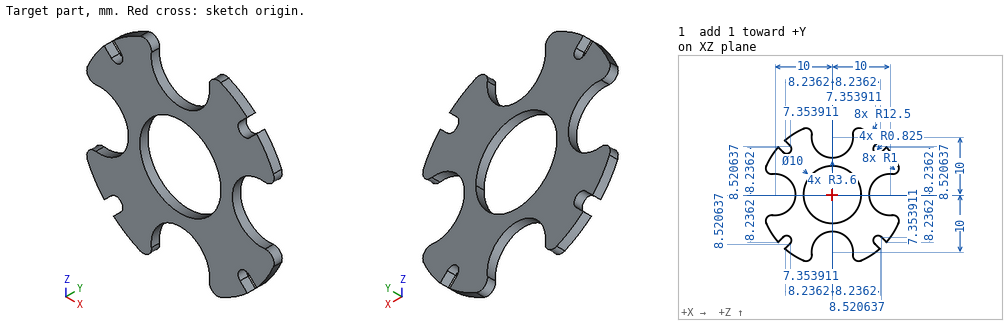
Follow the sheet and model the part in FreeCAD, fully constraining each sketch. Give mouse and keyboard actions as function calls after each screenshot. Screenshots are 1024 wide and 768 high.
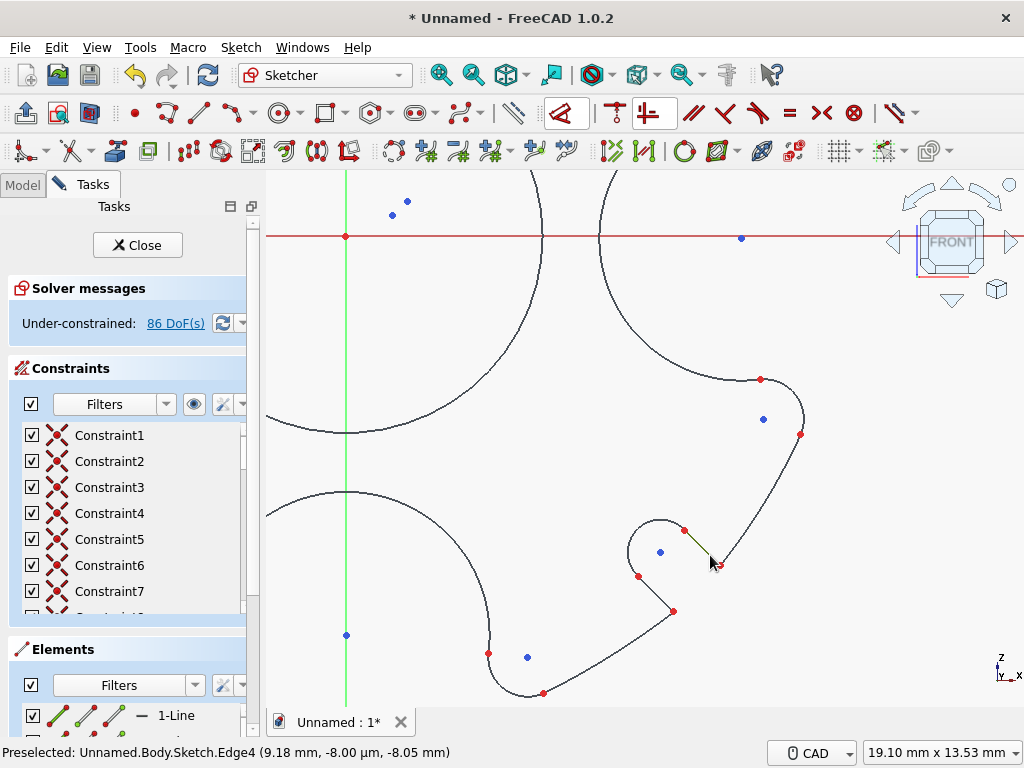
click(656, 520)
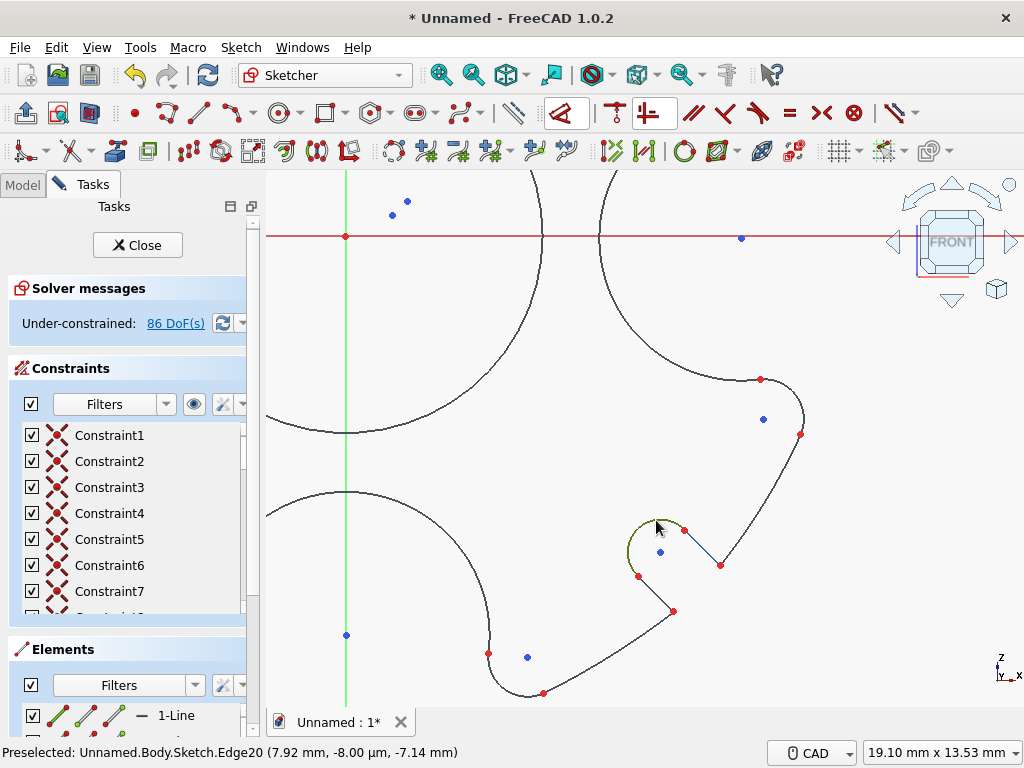
click(758, 114)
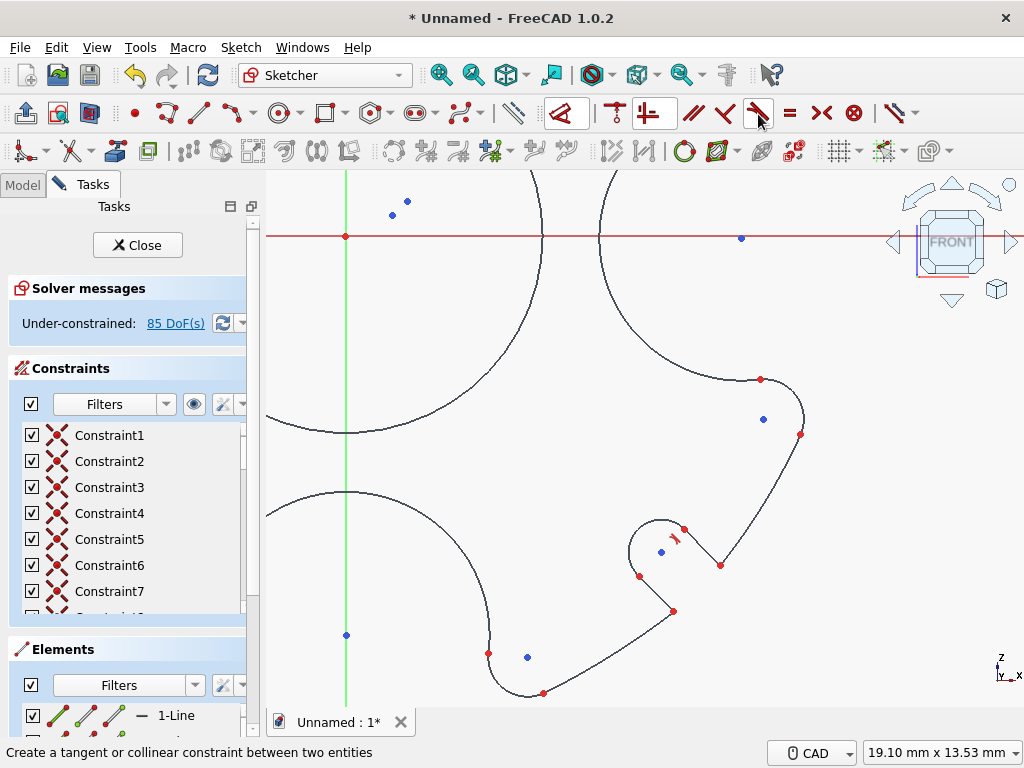
click(650, 587)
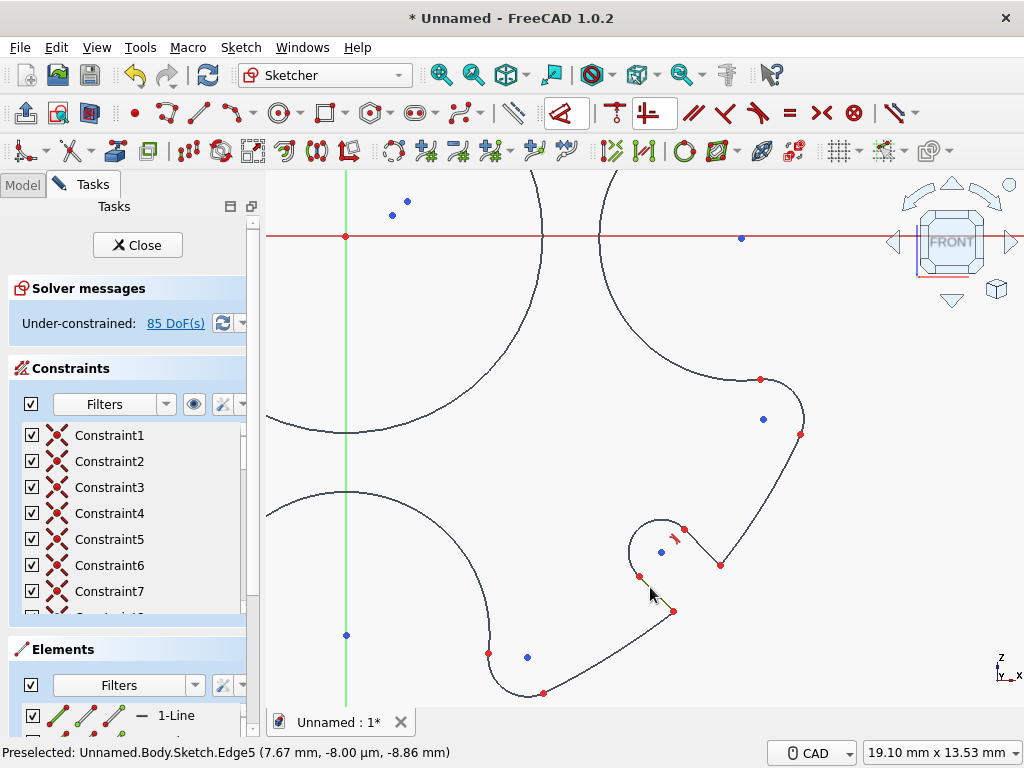
click(656, 520)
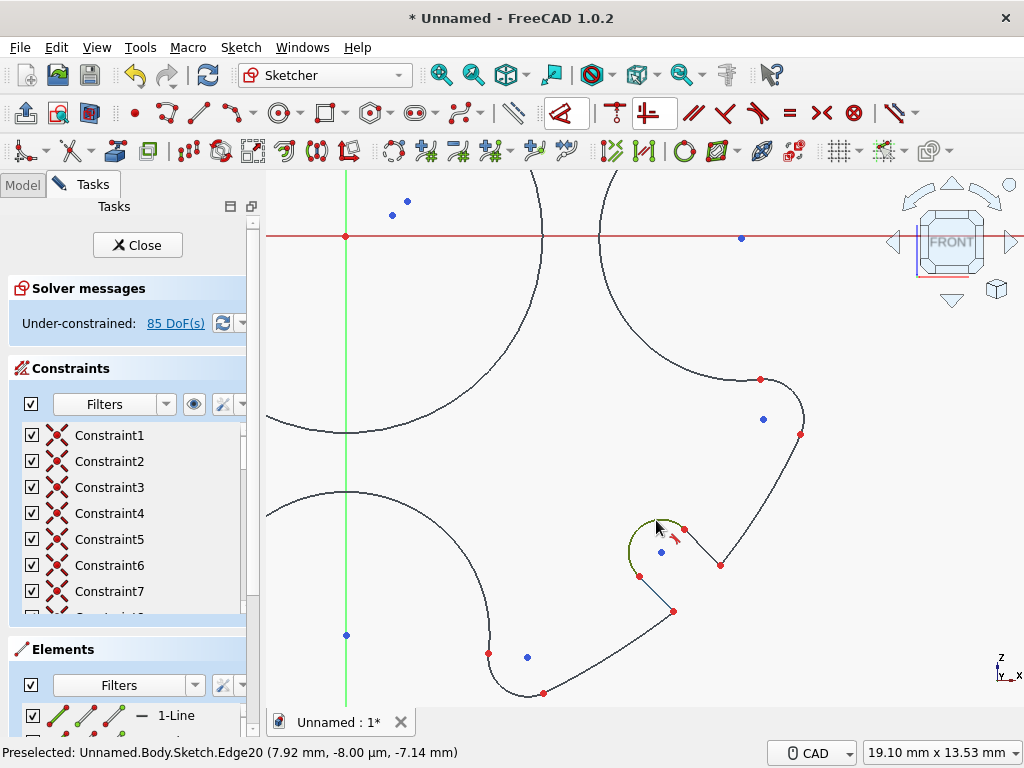
key(t)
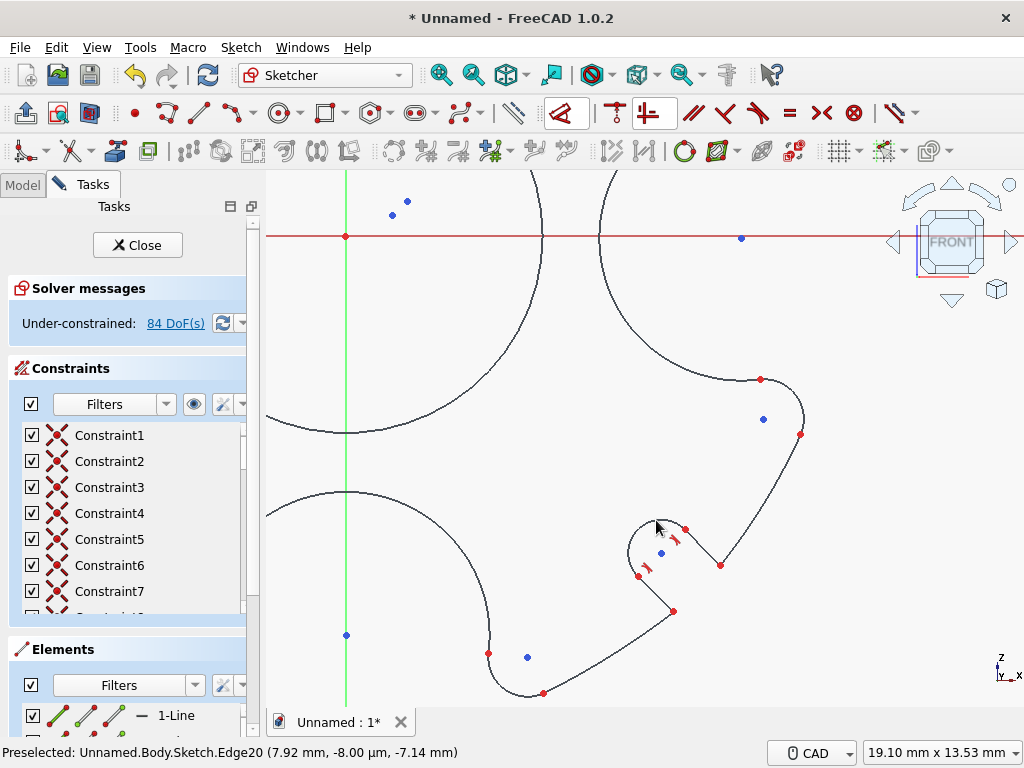
scroll(711, 556, down, 5)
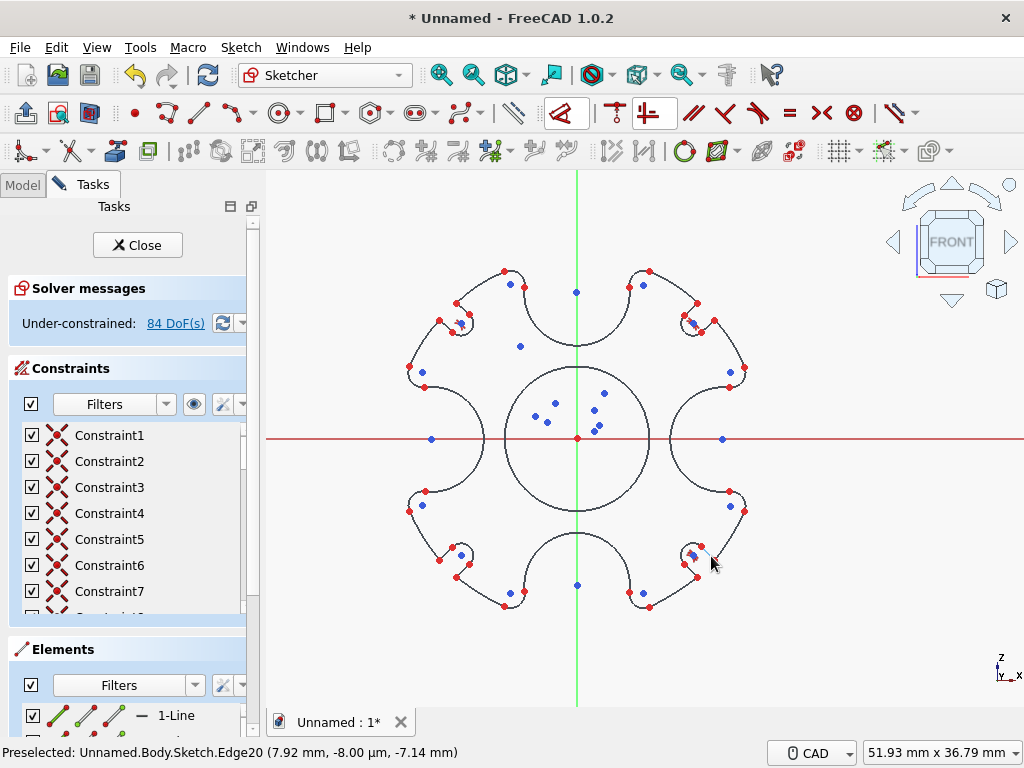
scroll(461, 573, up, 5)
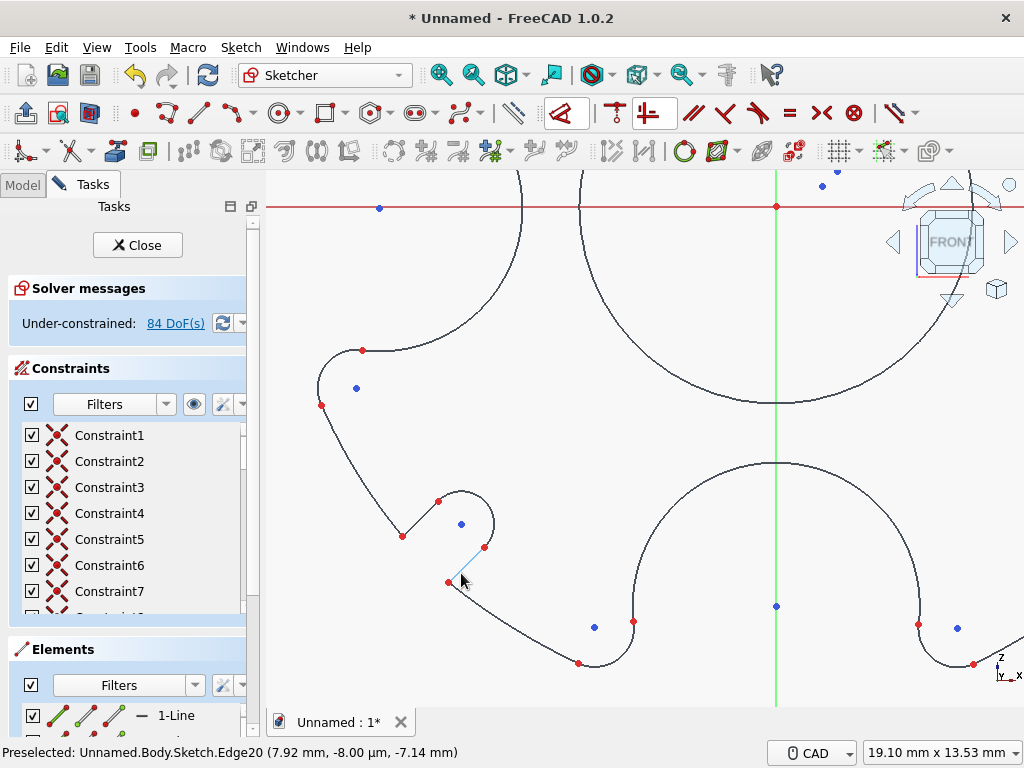
click(460, 572)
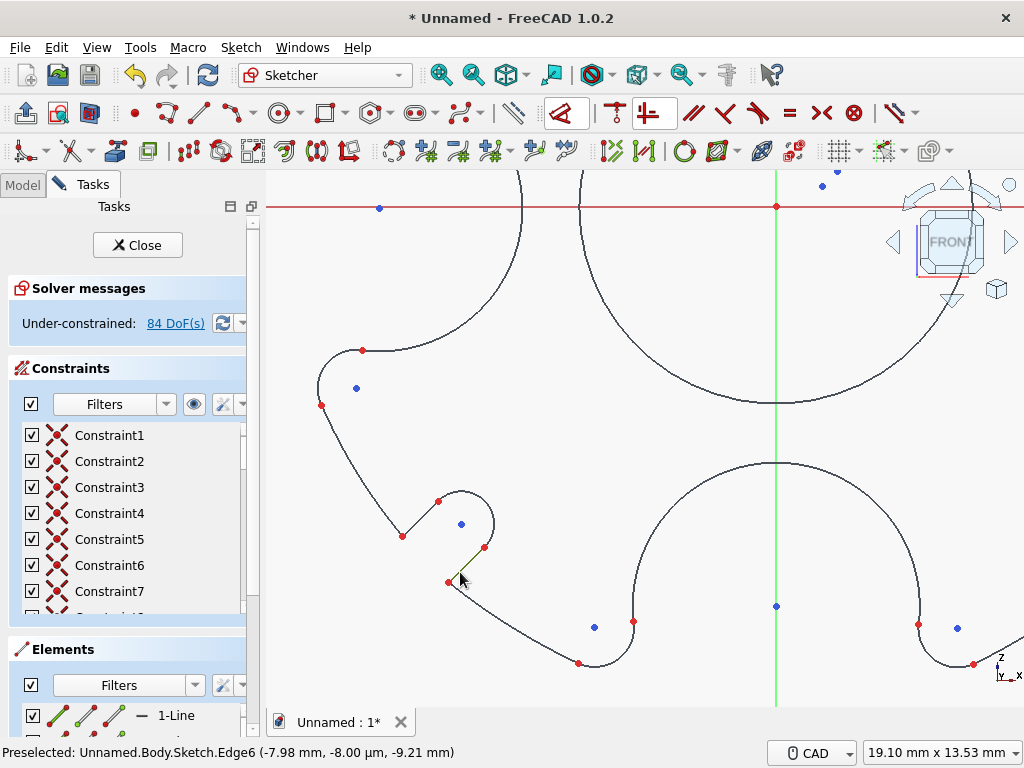
click(494, 519)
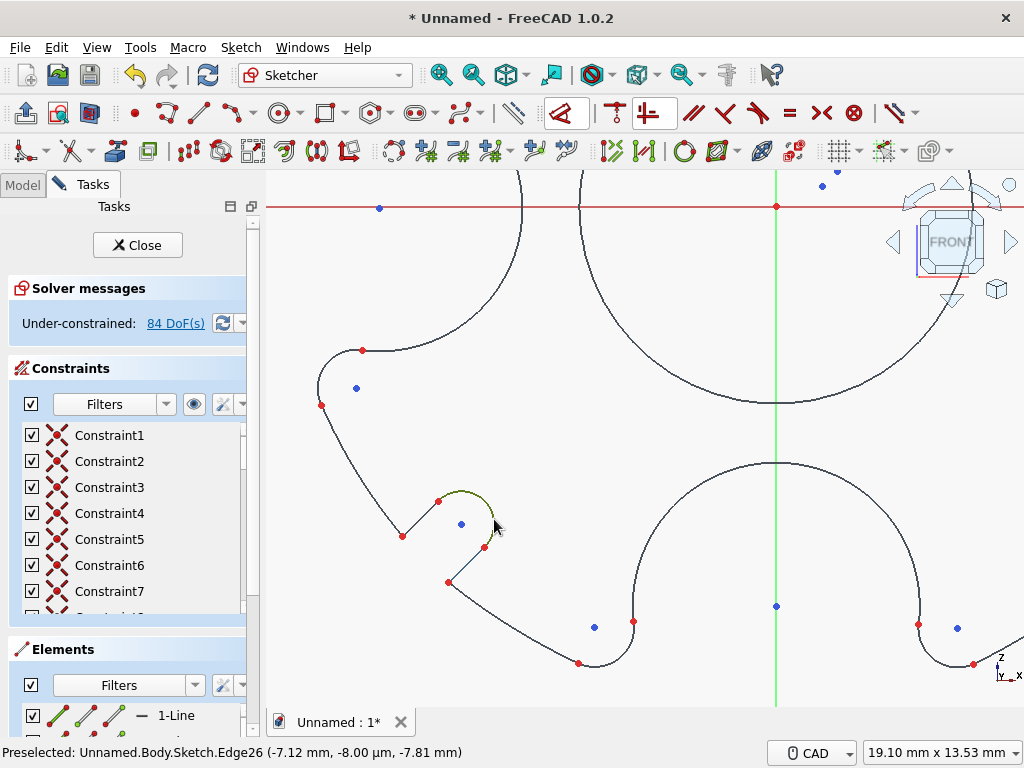
click(758, 114)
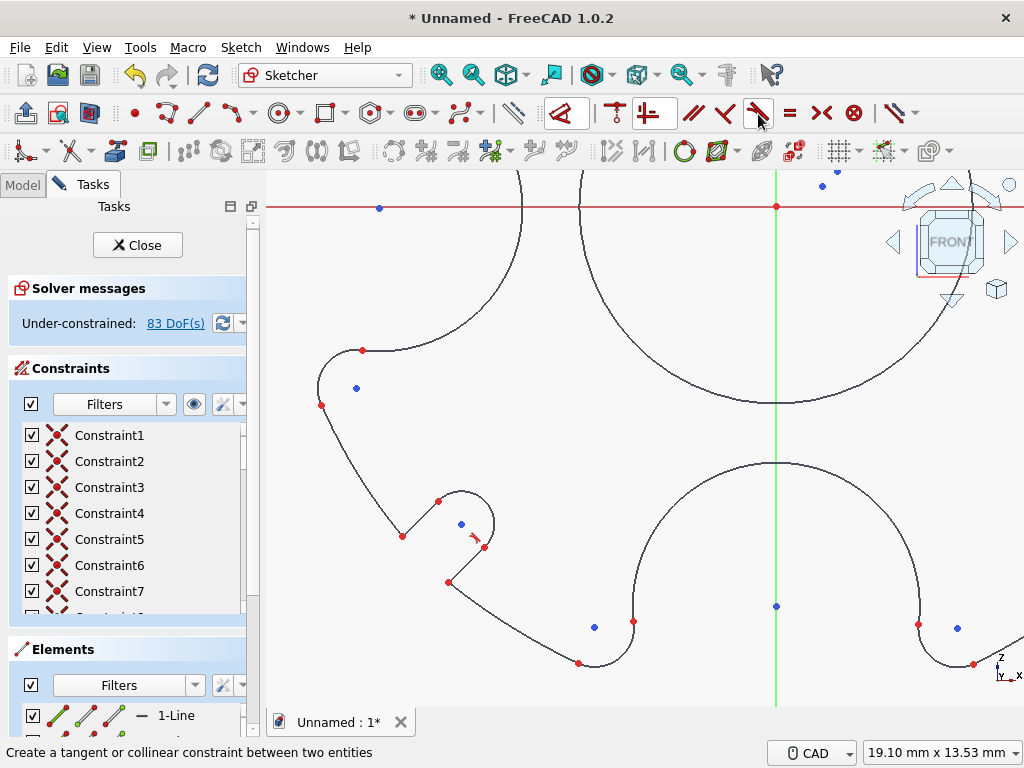
click(428, 512)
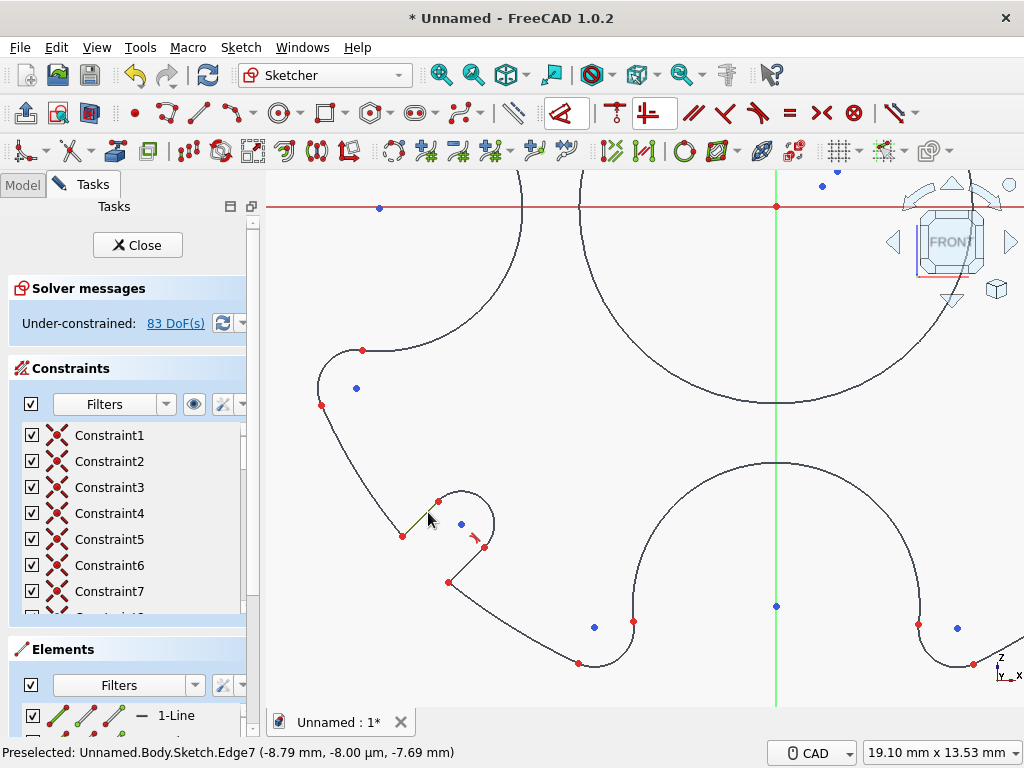
click(494, 519)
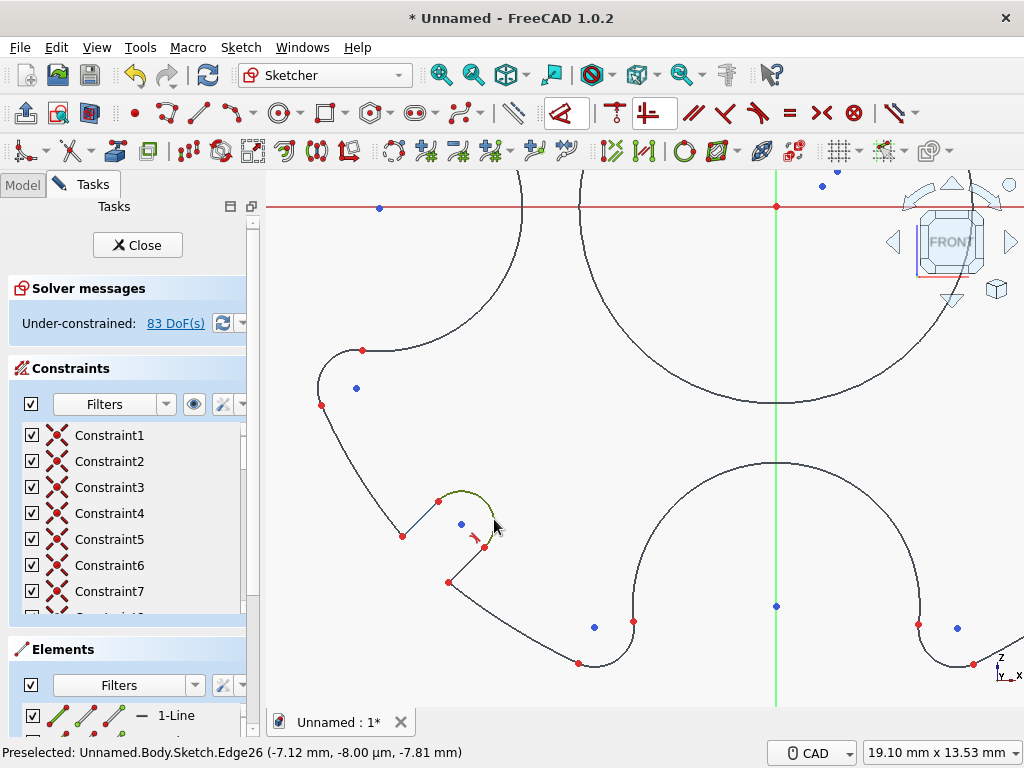
click(758, 114)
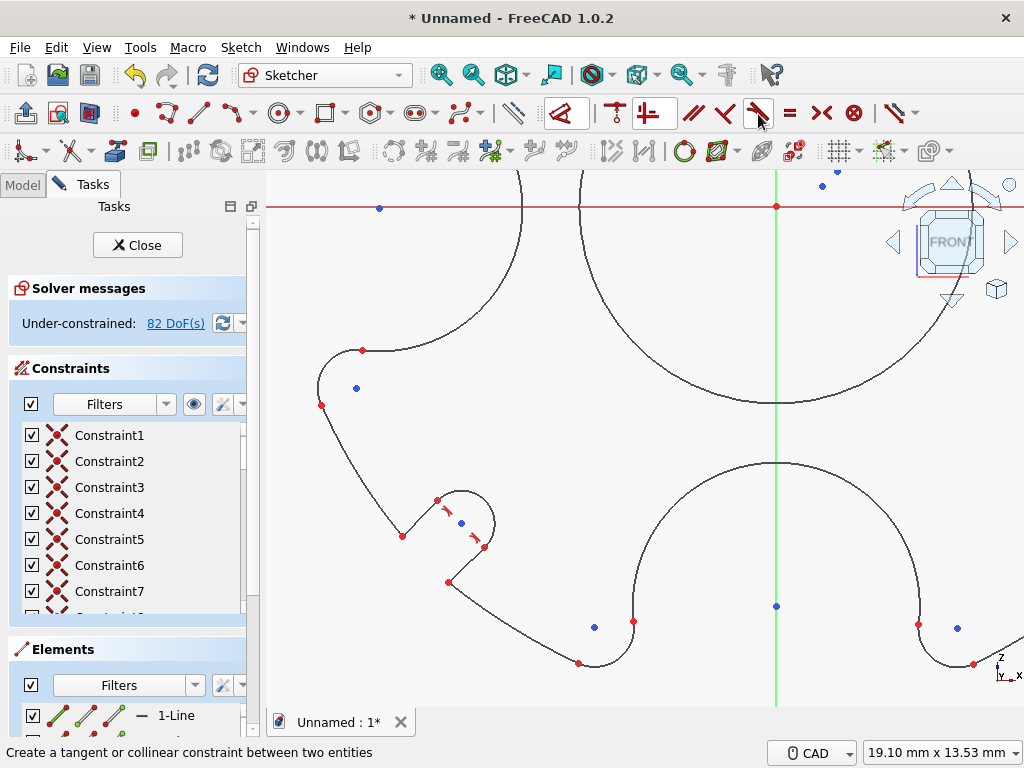
scroll(460, 573, down, 5)